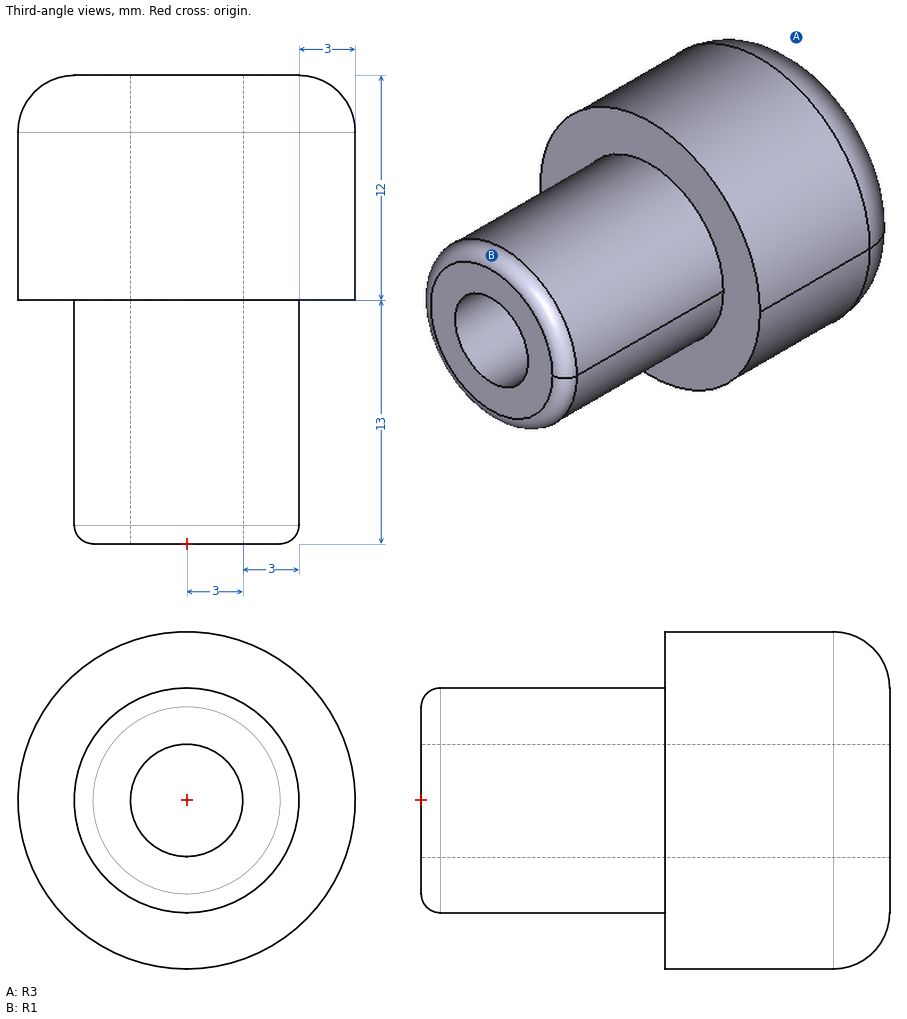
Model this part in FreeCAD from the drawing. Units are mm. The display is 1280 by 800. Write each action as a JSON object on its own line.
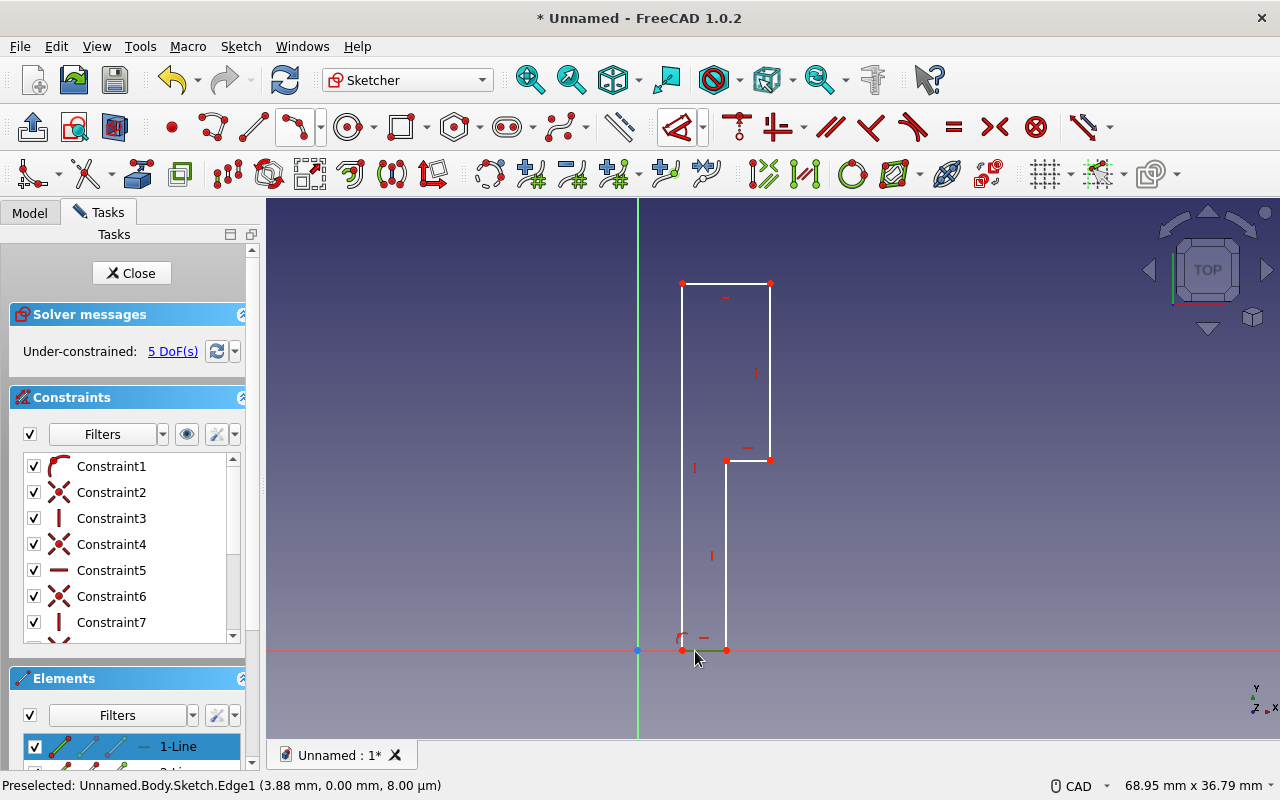
{"action": "key", "text": "l"}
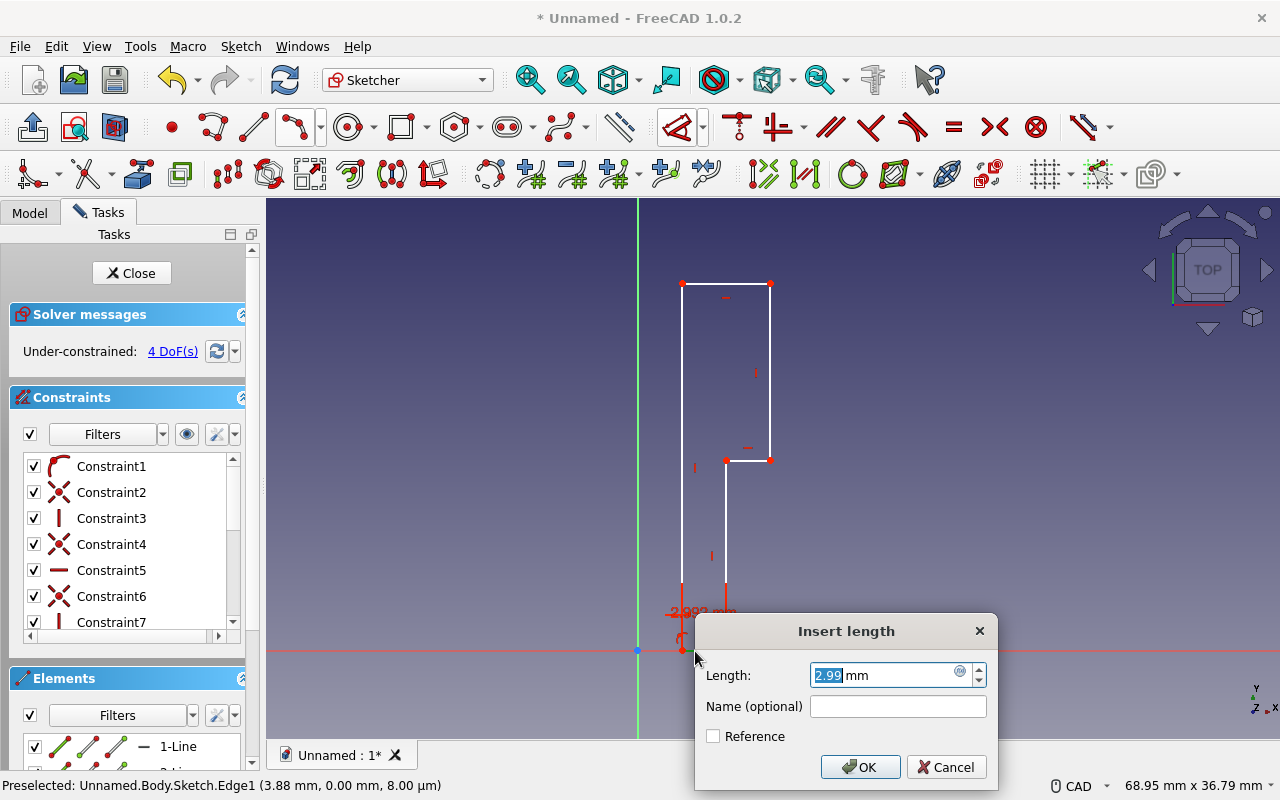
{"action": "type", "text": "3"}
{"action": "key", "text": "Return"}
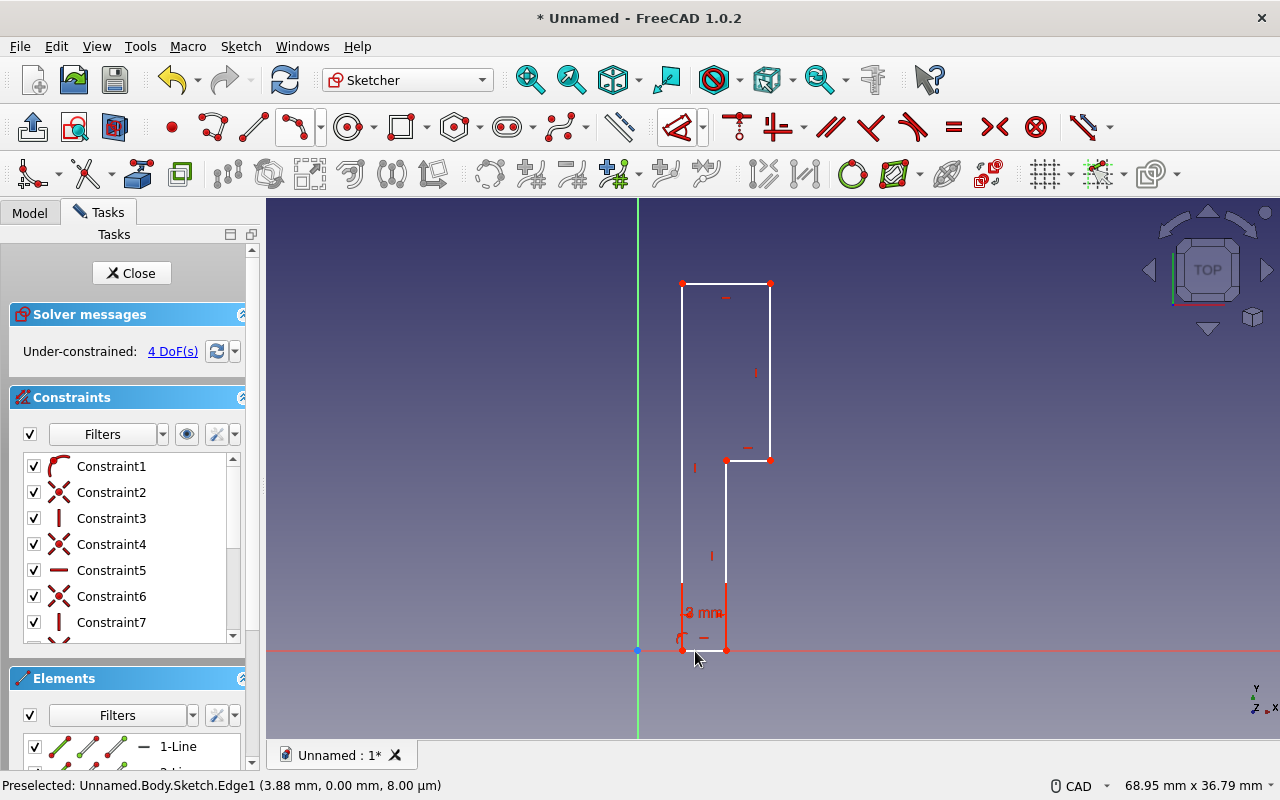
{"action": "left_click", "coordinate": [739, 461]}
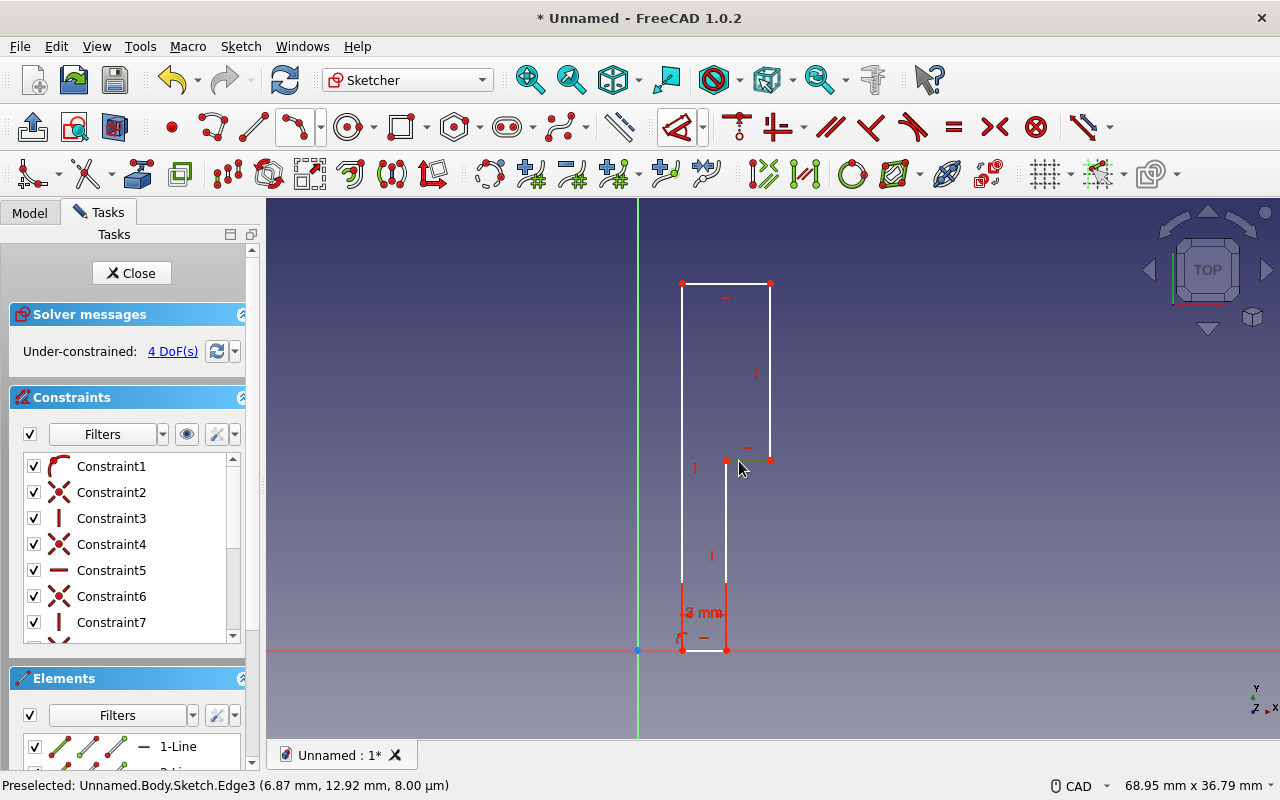
{"action": "key", "text": "l"}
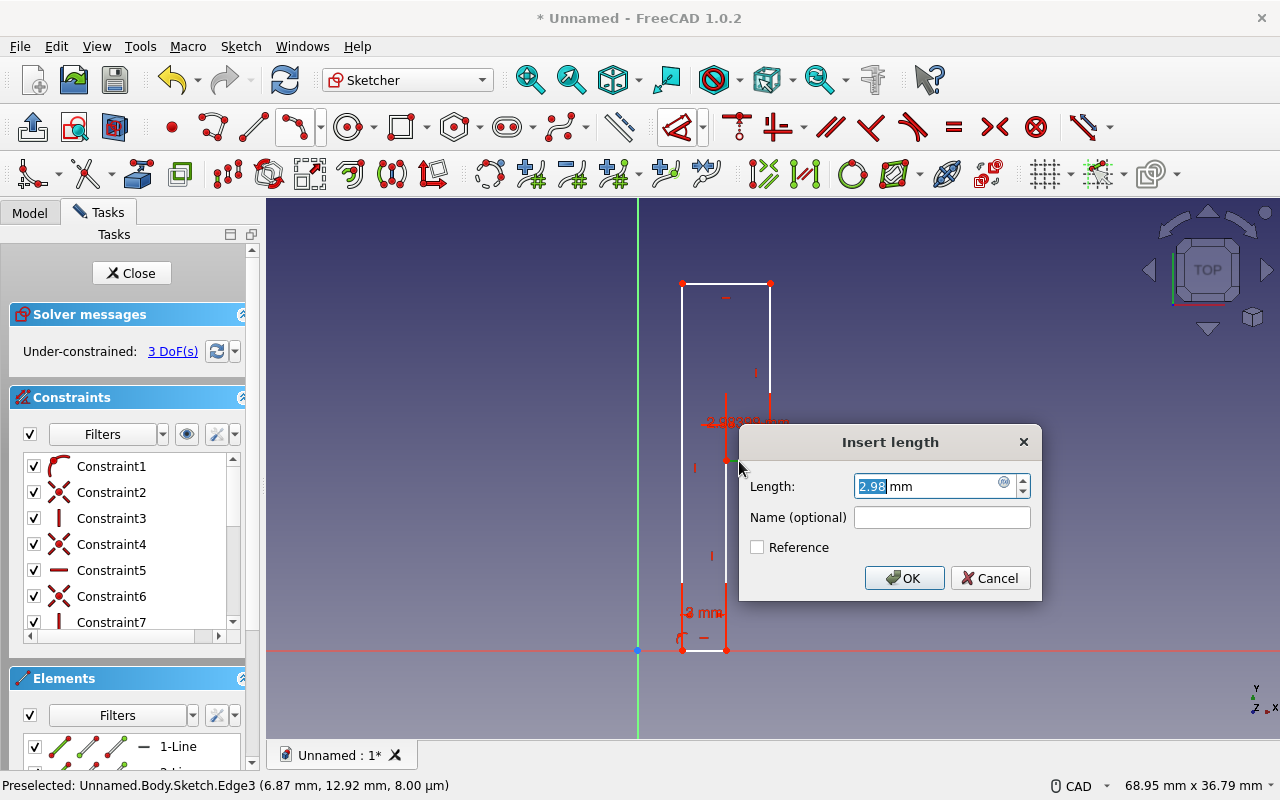
{"action": "type", "text": "3"}
{"action": "key", "text": "Return"}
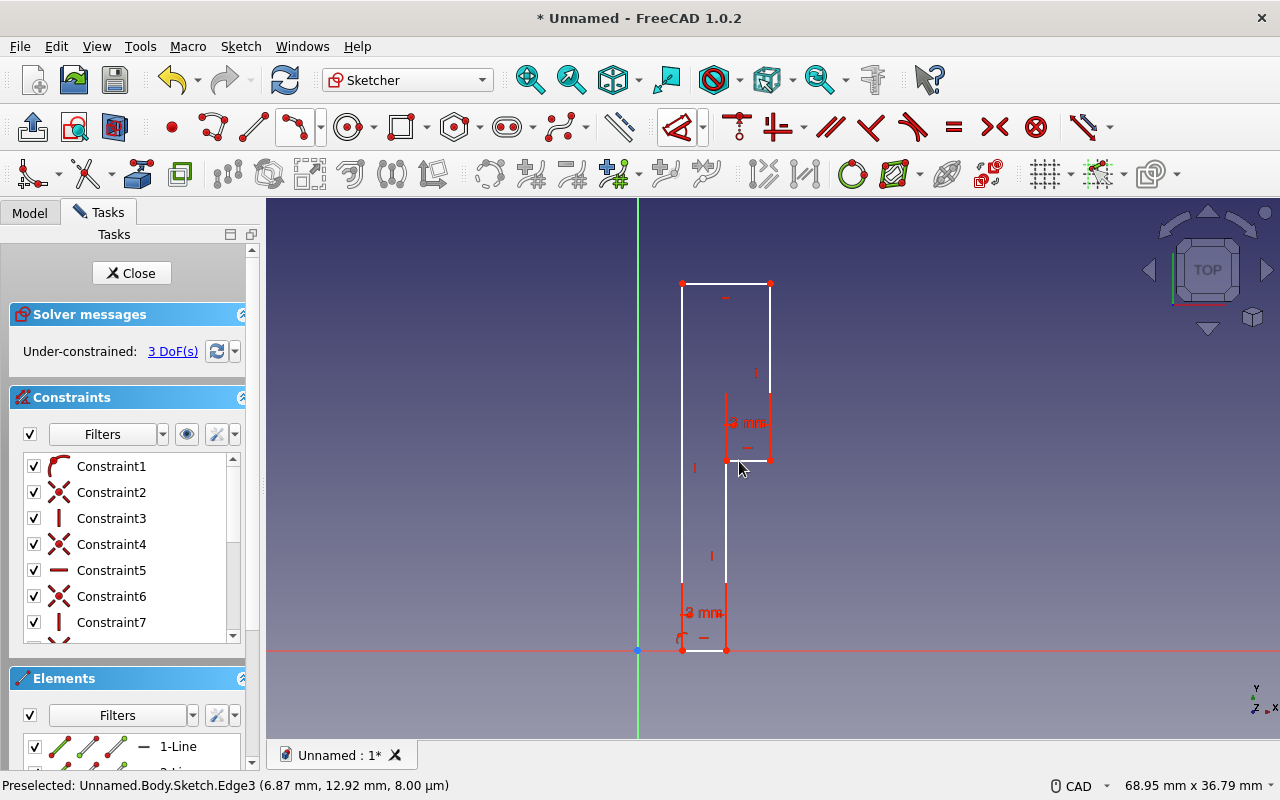
{"action": "left_click", "coordinate": [726, 594]}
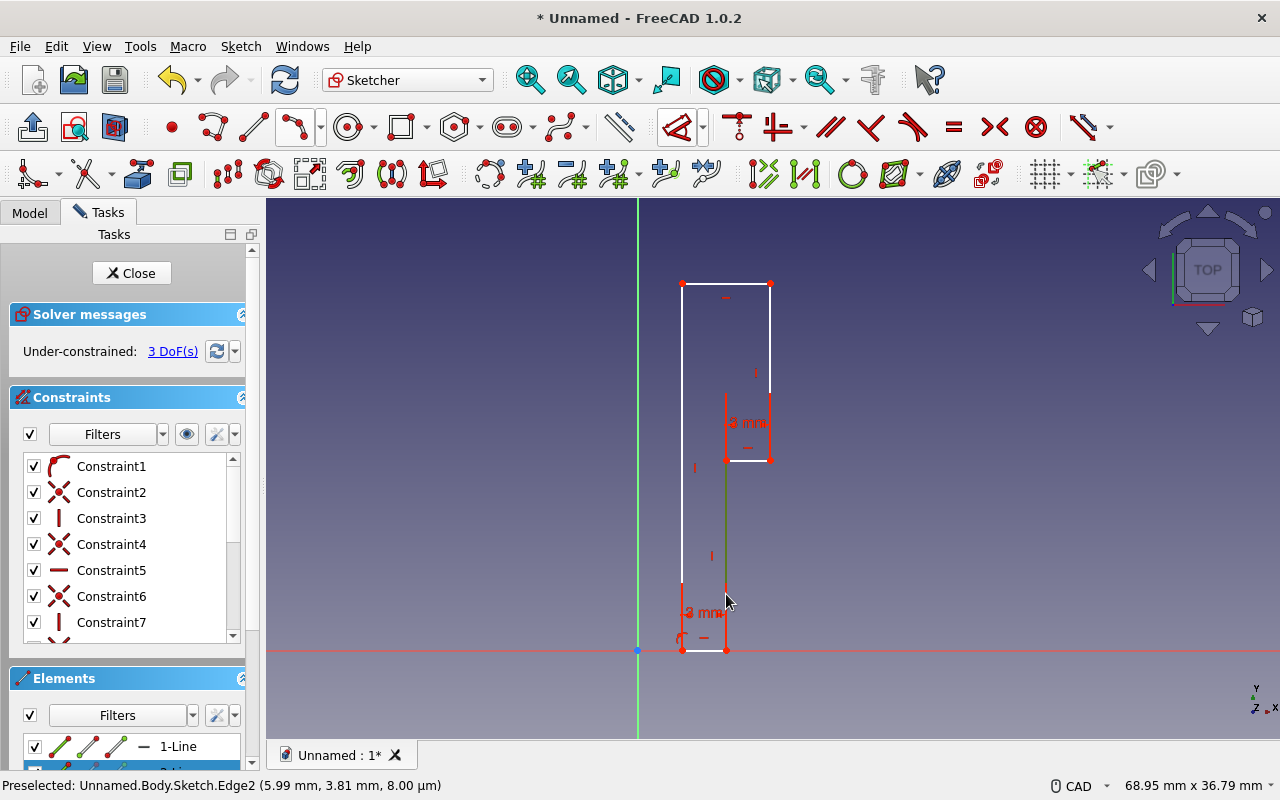
{"action": "key", "text": "i"}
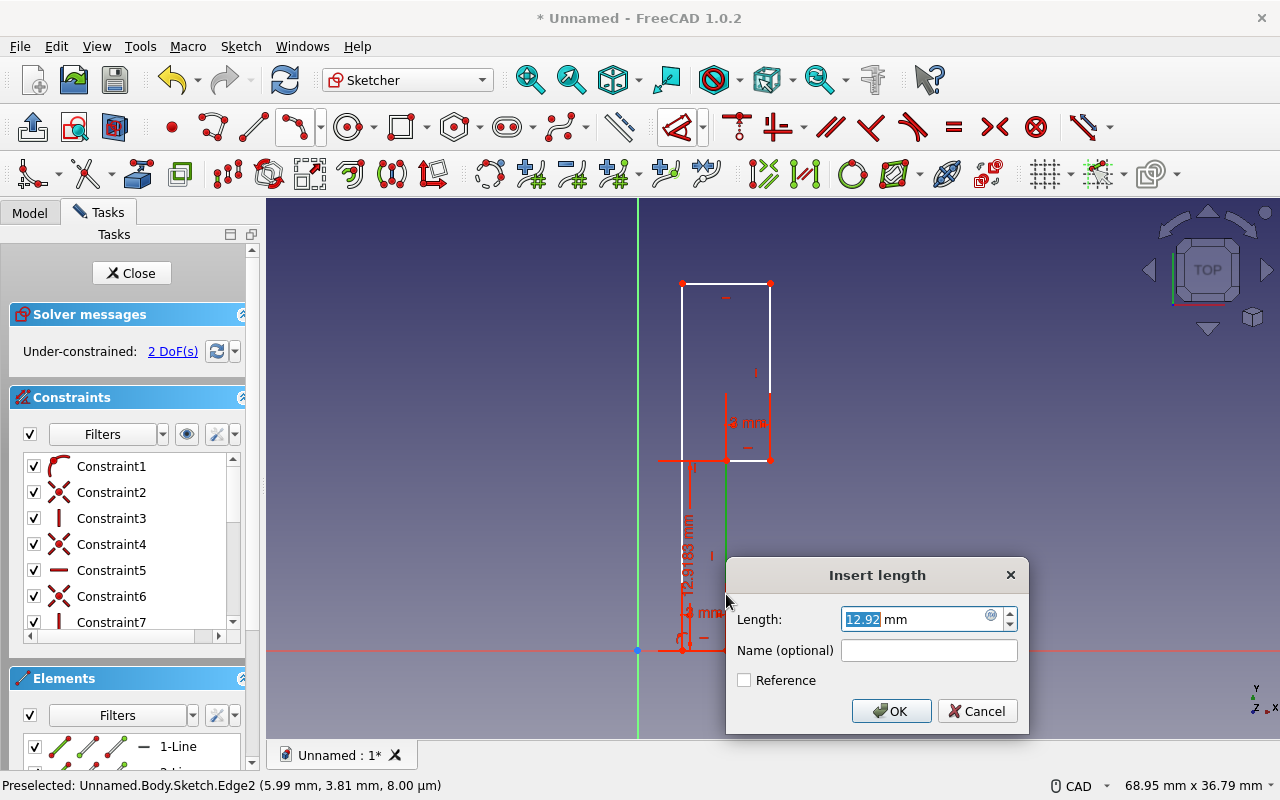
{"action": "type", "text": "13"}
{"action": "key", "text": "Return"}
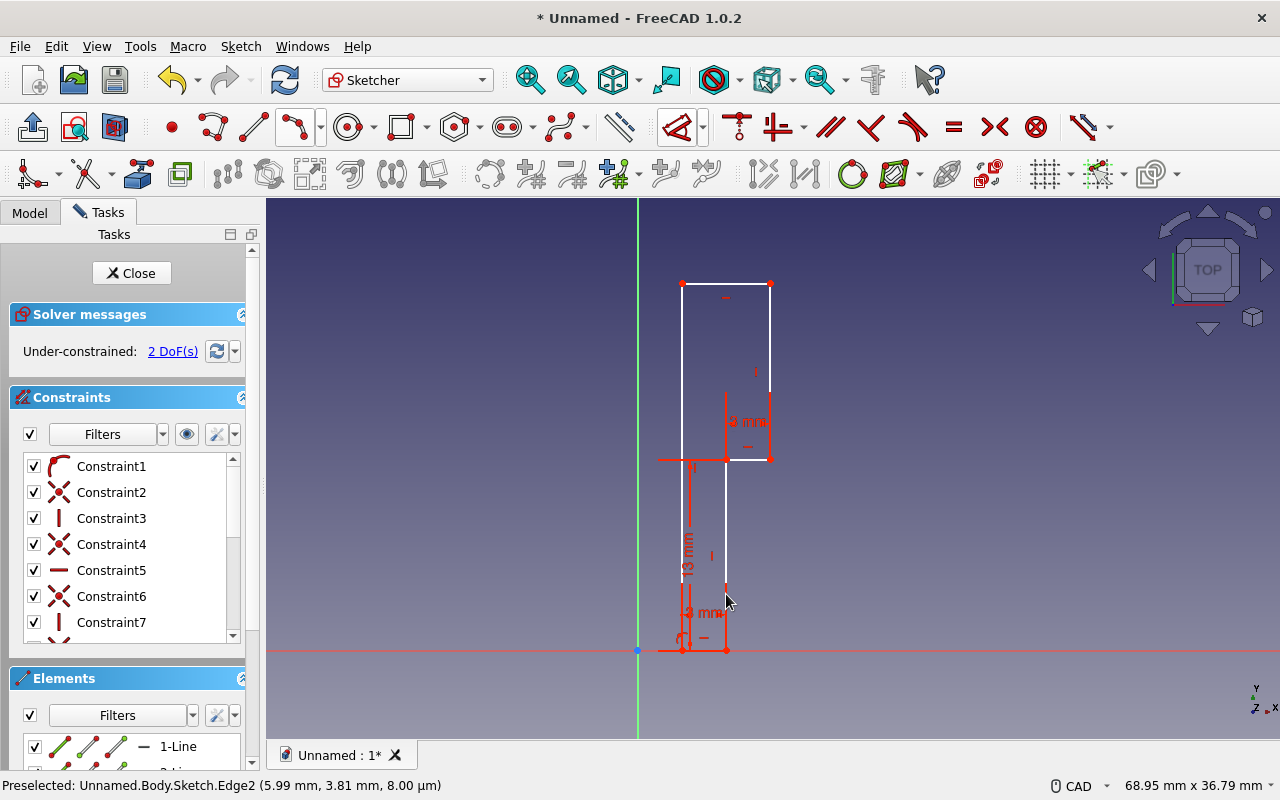
{"action": "left_click", "coordinate": [770, 407]}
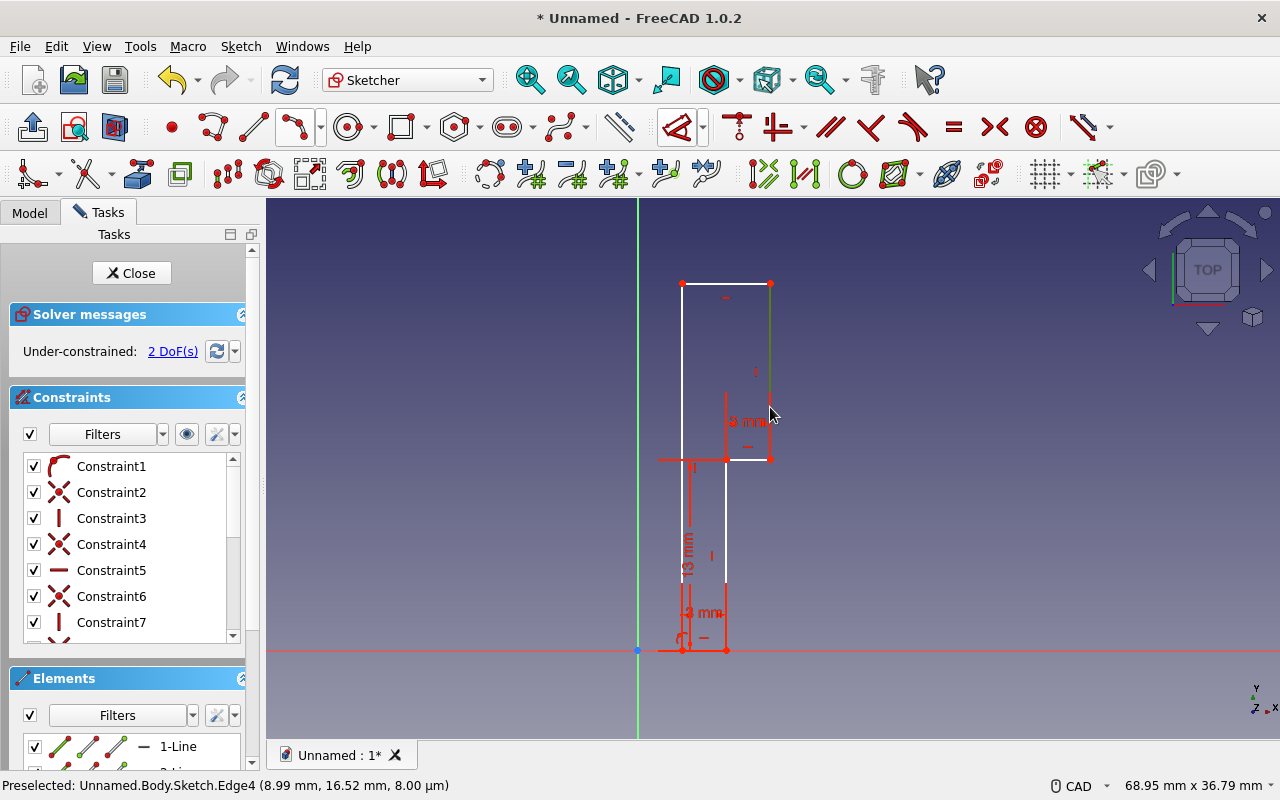
{"action": "key", "text": "i"}